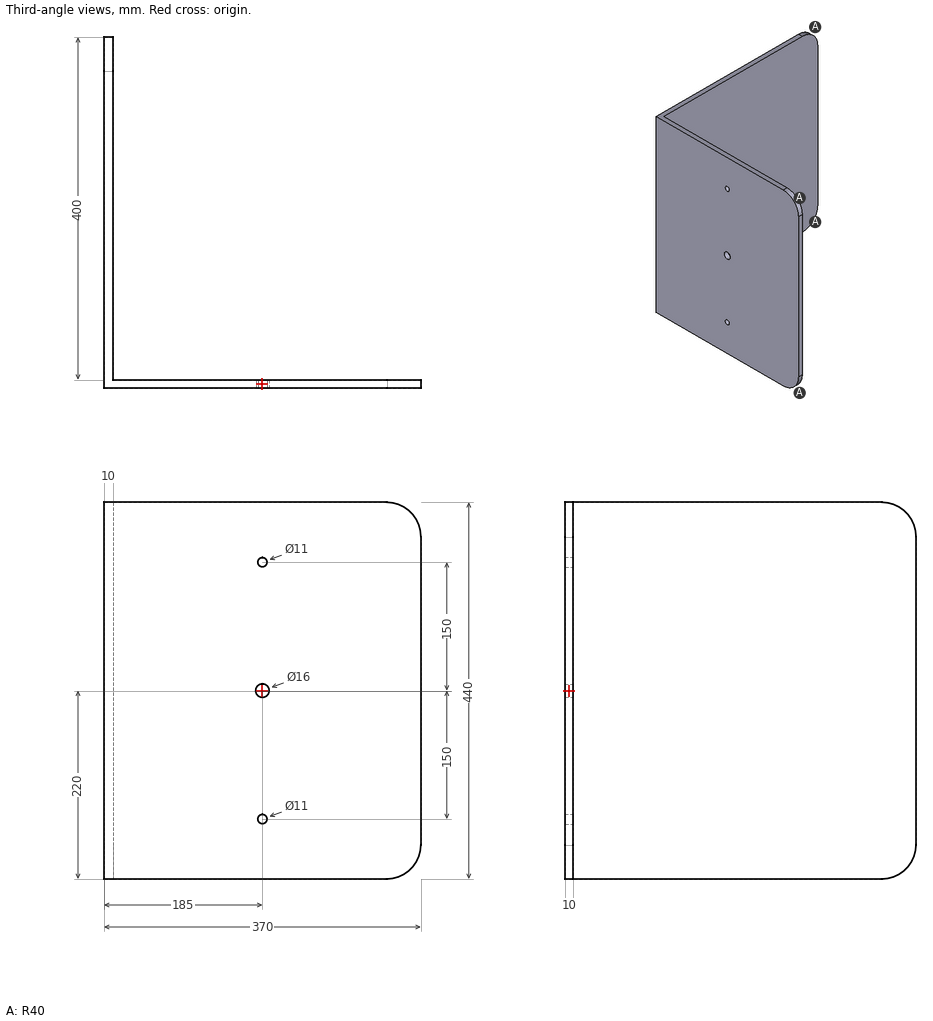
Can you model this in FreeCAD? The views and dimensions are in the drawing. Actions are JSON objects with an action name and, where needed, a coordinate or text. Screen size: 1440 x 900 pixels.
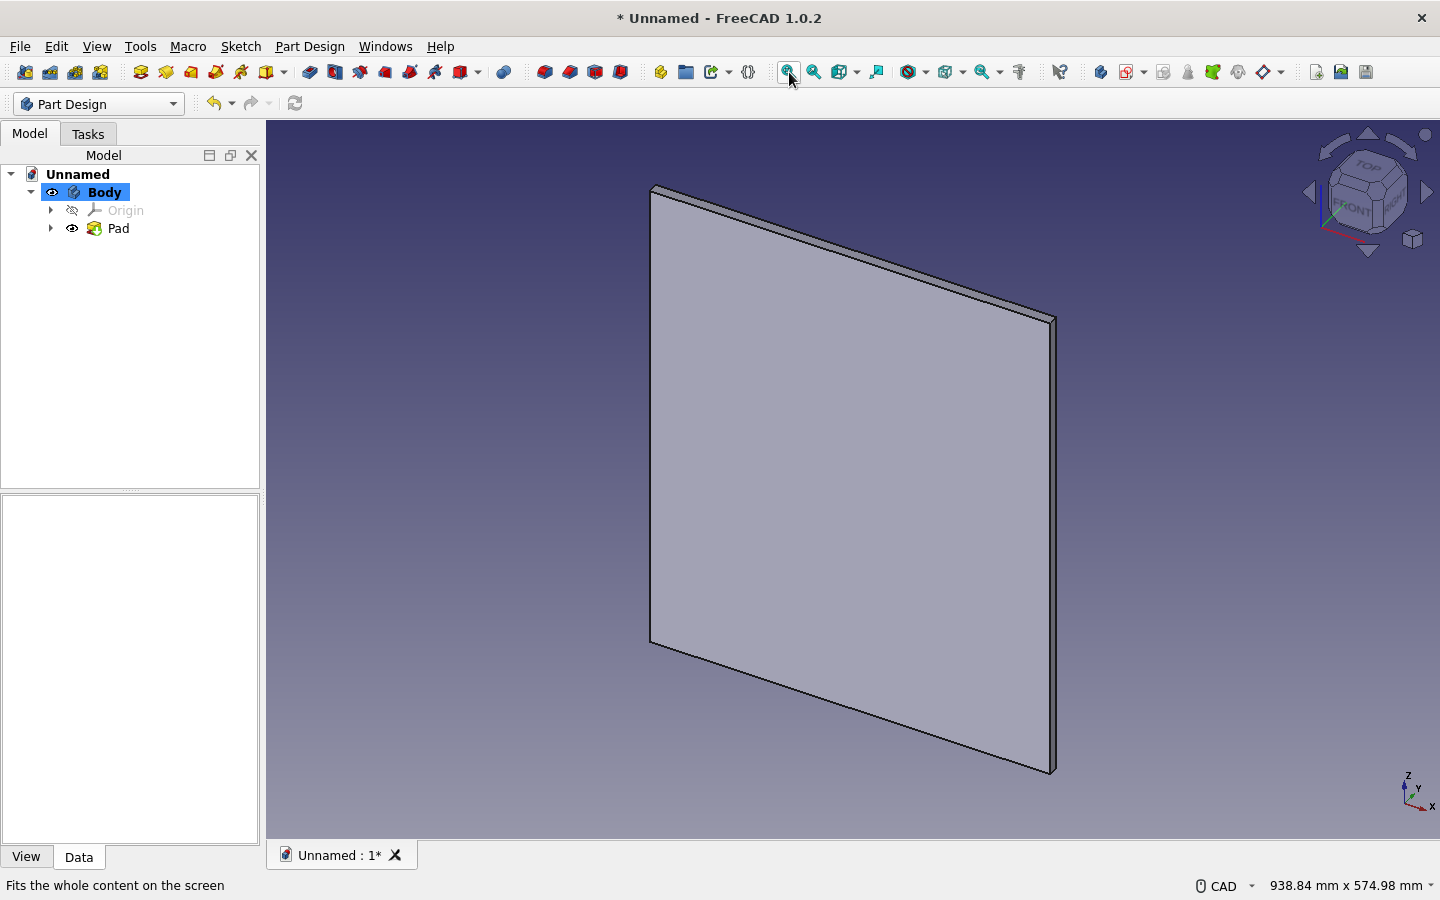
{"action": "key", "text": "4"}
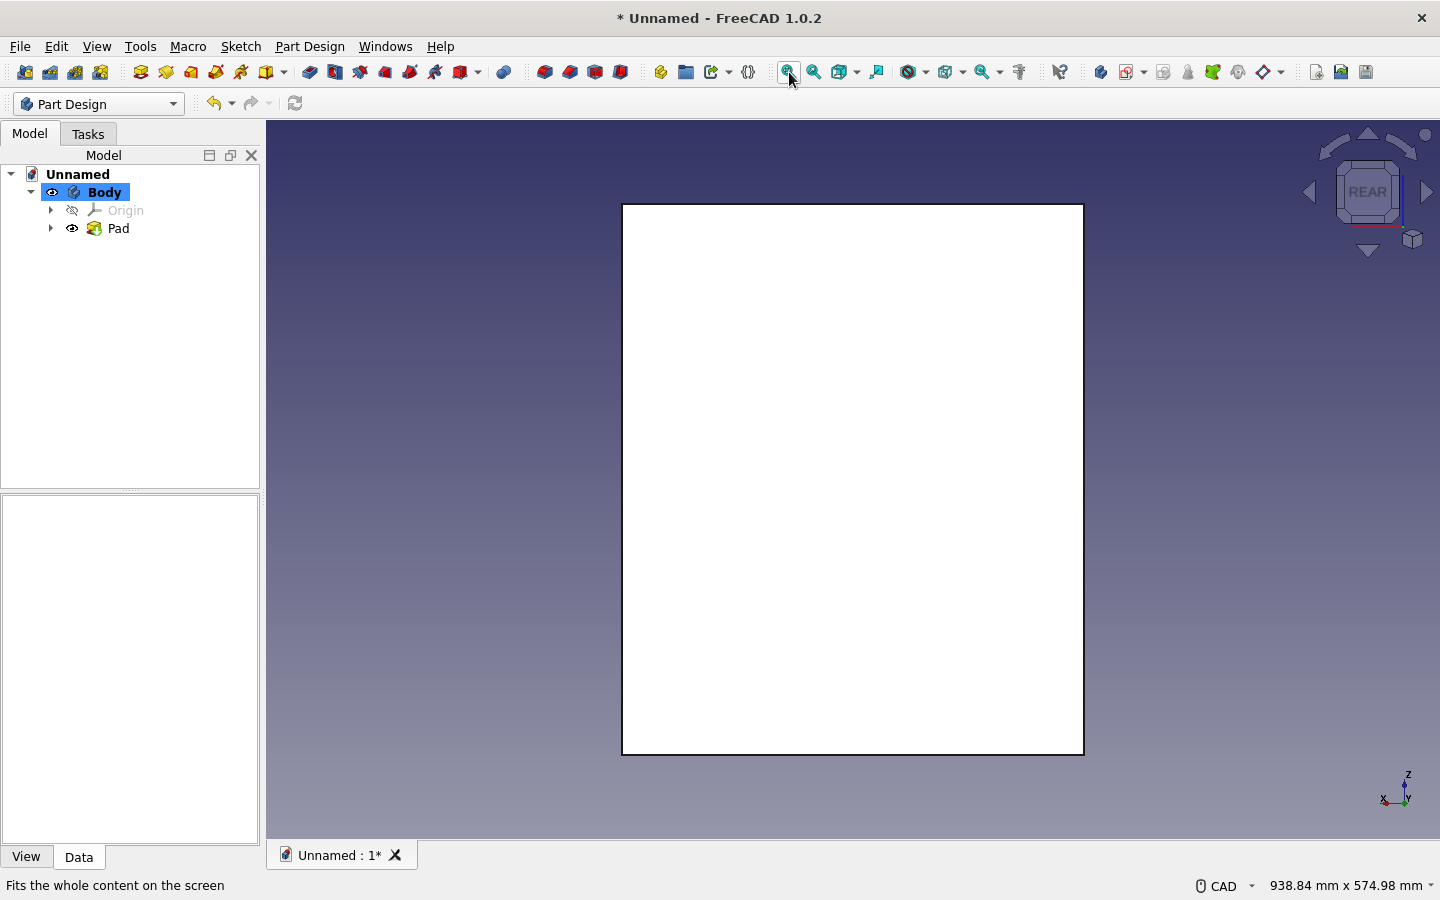
{"action": "left_click", "coordinate": [853, 478]}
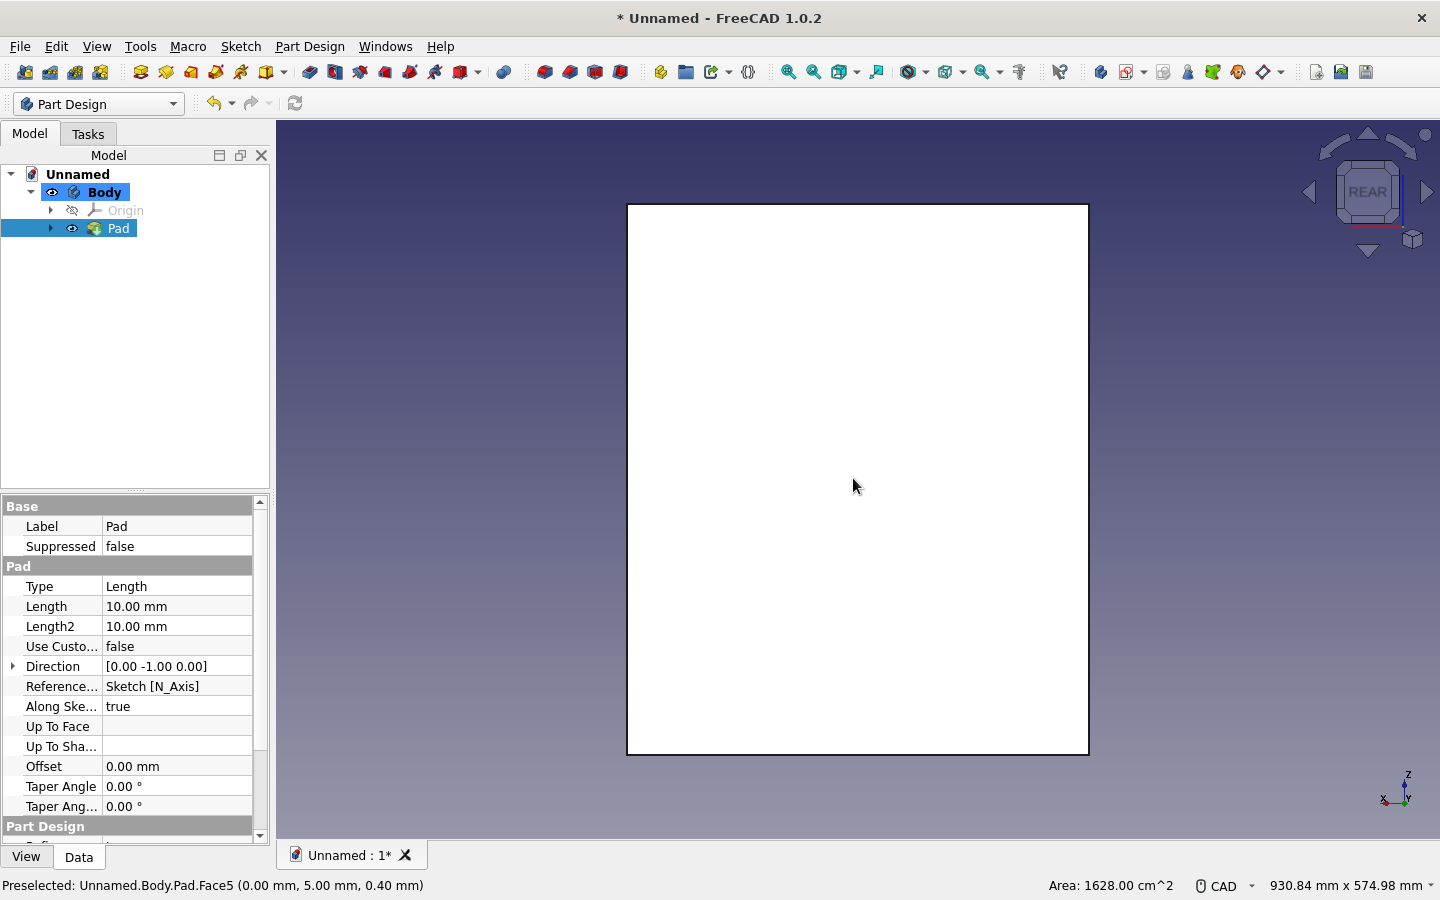
{"action": "left_click", "coordinate": [1126, 72]}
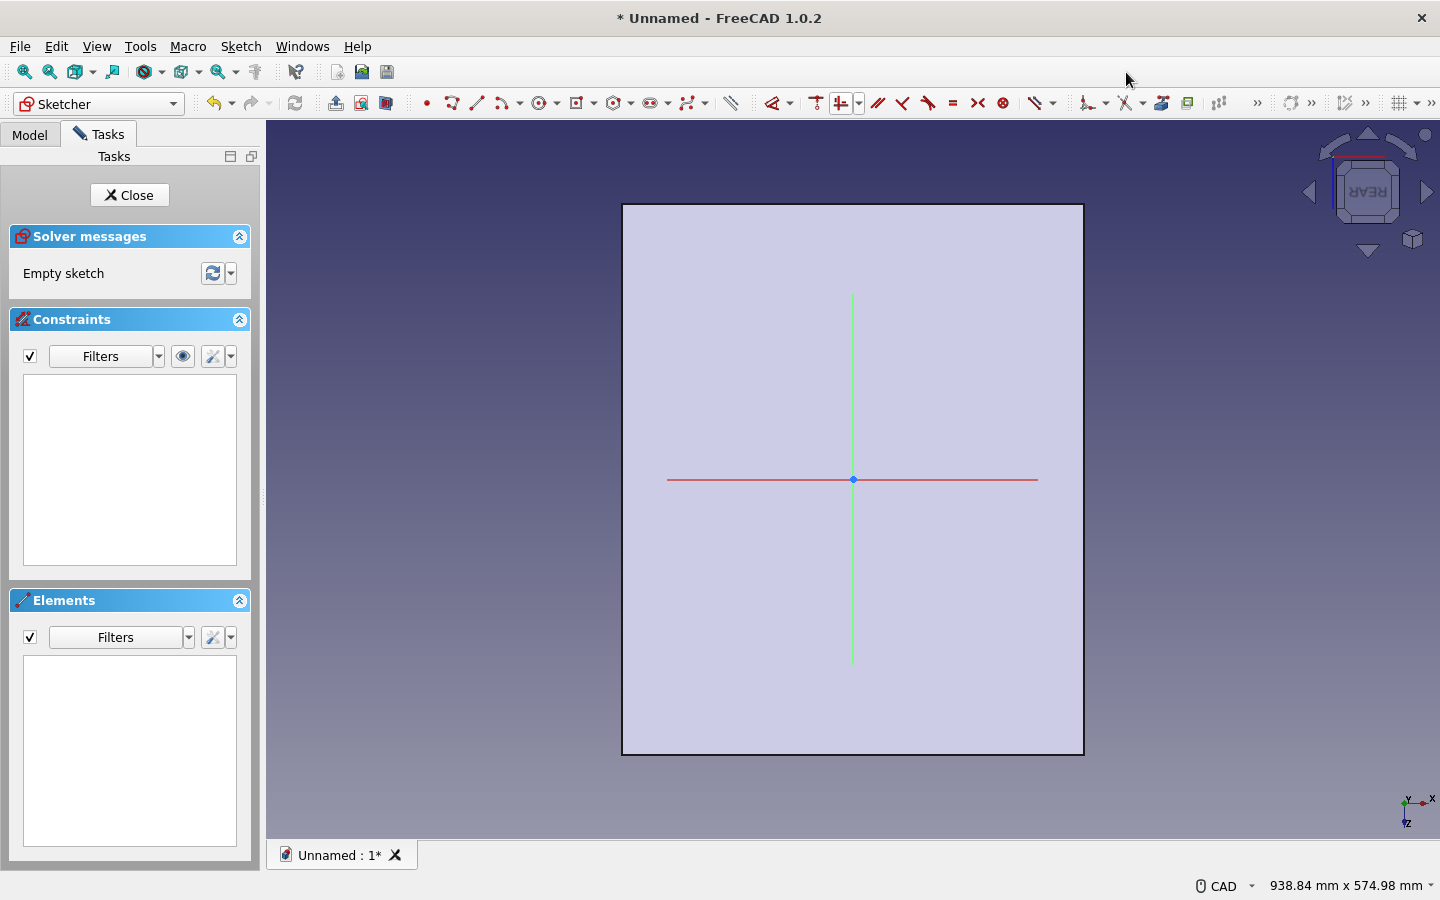
{"action": "scroll", "coordinate": [857, 480], "scroll_direction": "up", "scroll_amount": 15}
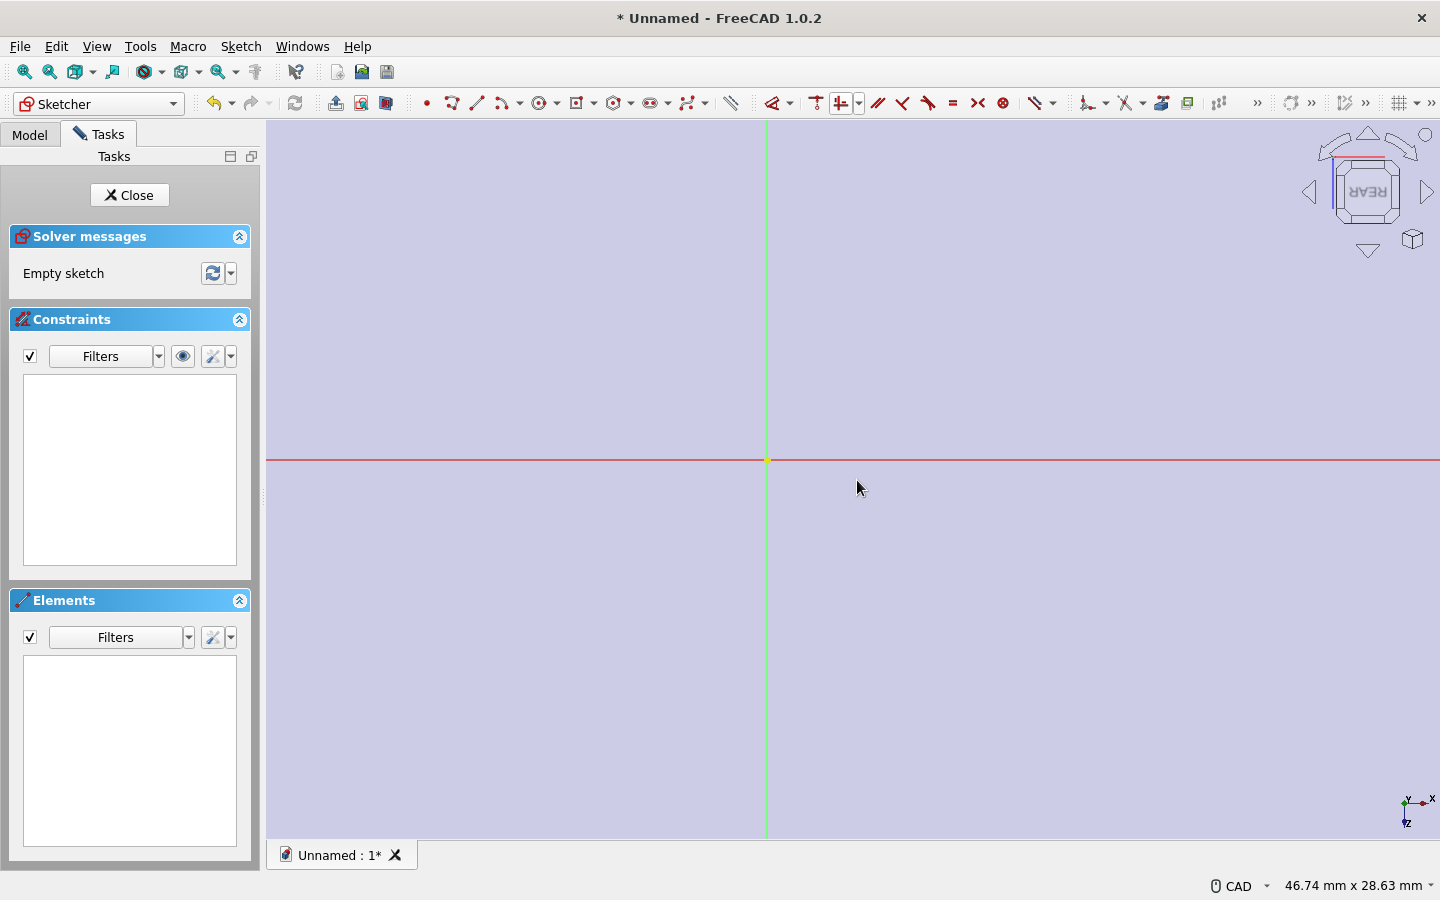
{"action": "left_click", "coordinate": [538, 104]}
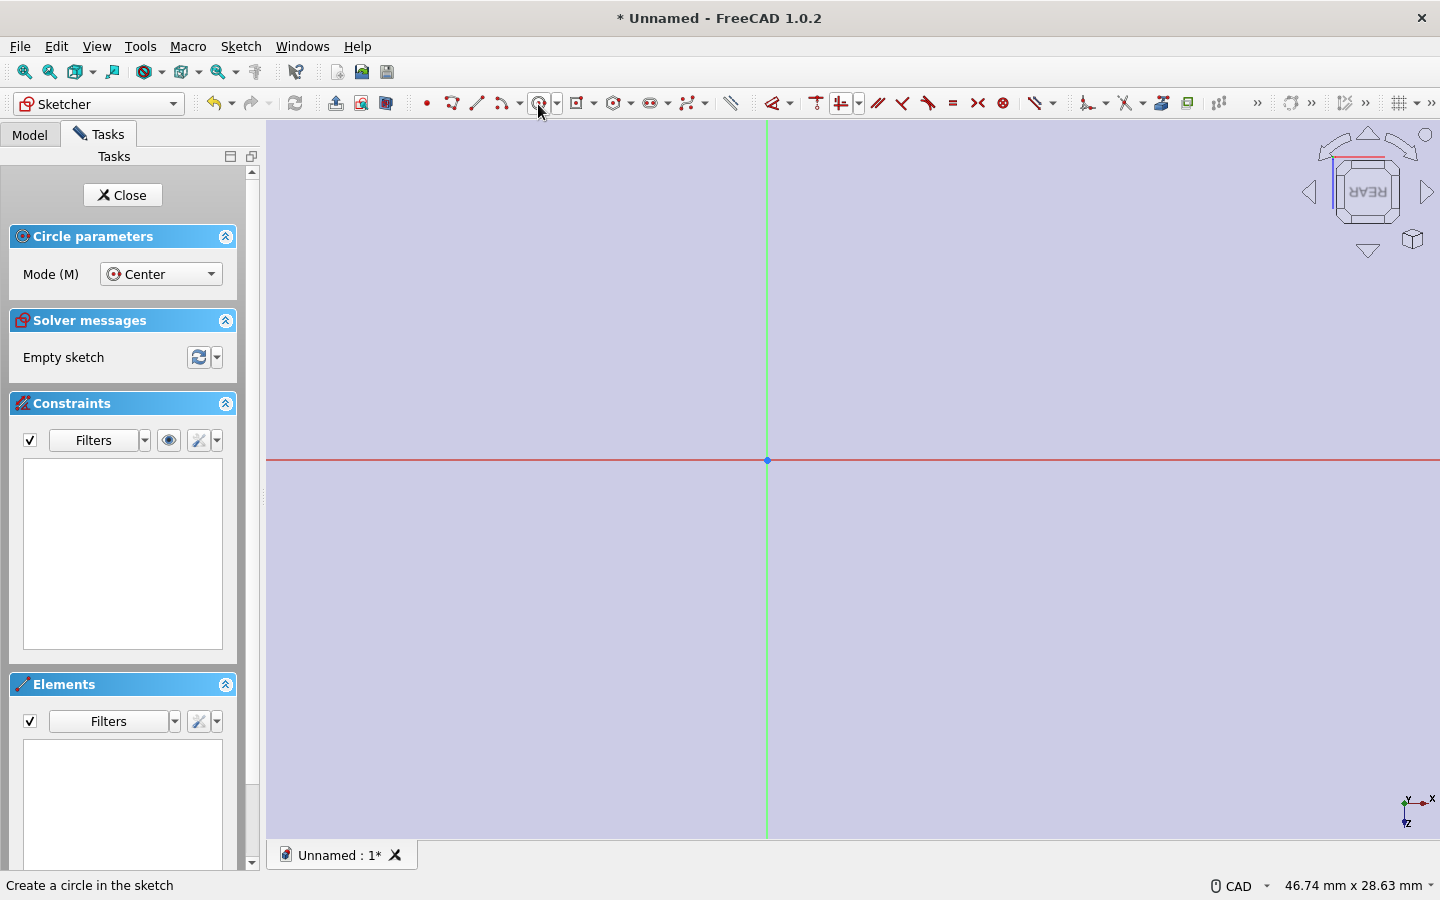
{"action": "left_click", "coordinate": [767, 460]}
{"action": "mouse_move", "coordinate": [909, 318]}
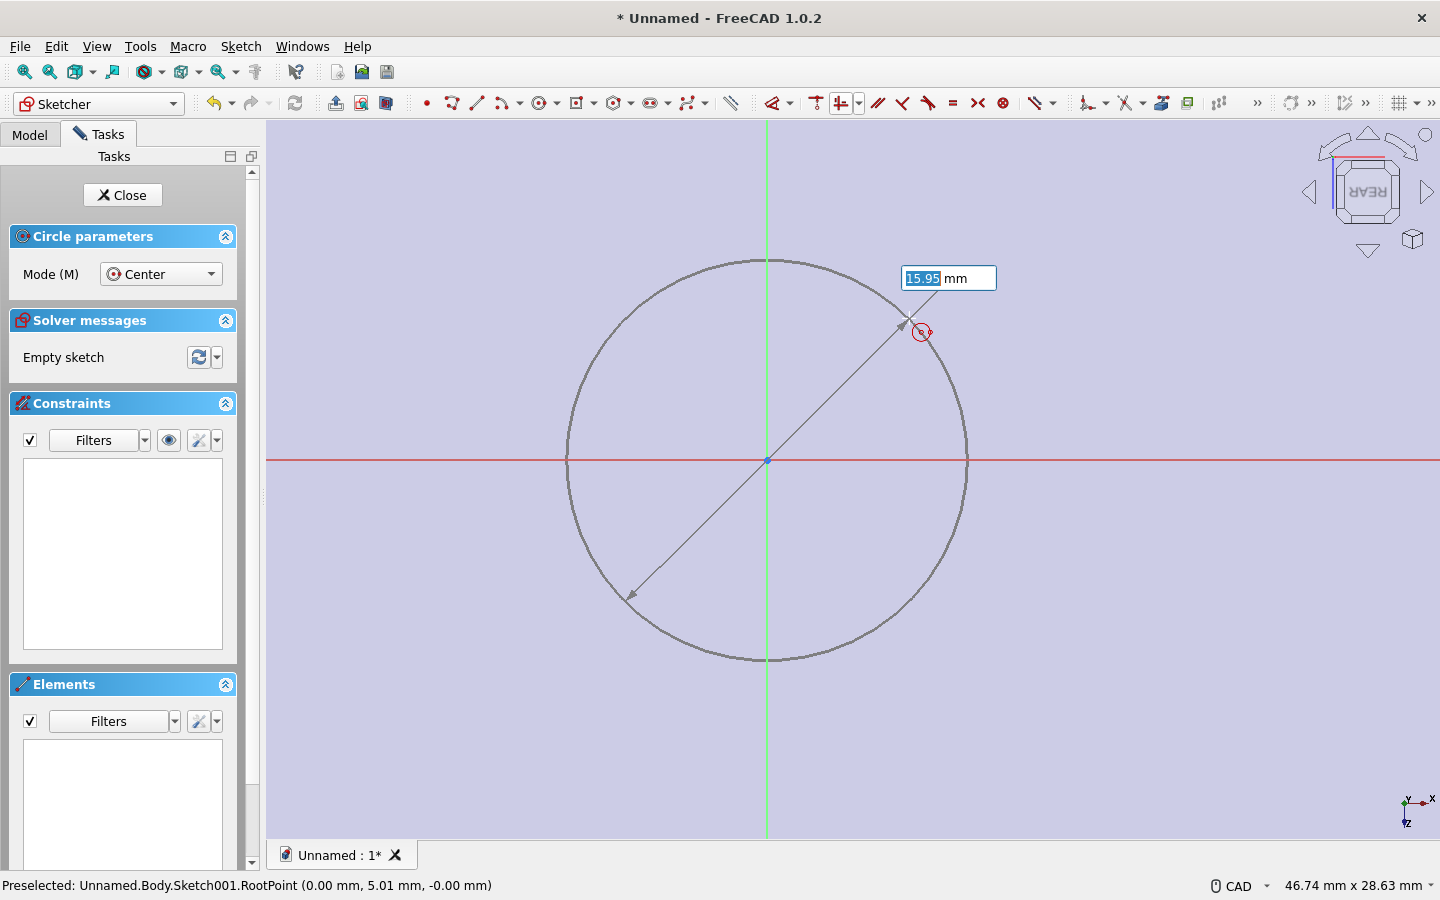
{"action": "type", "text": "16"}
{"action": "key", "text": "Return"}
{"action": "key", "text": "Escape"}